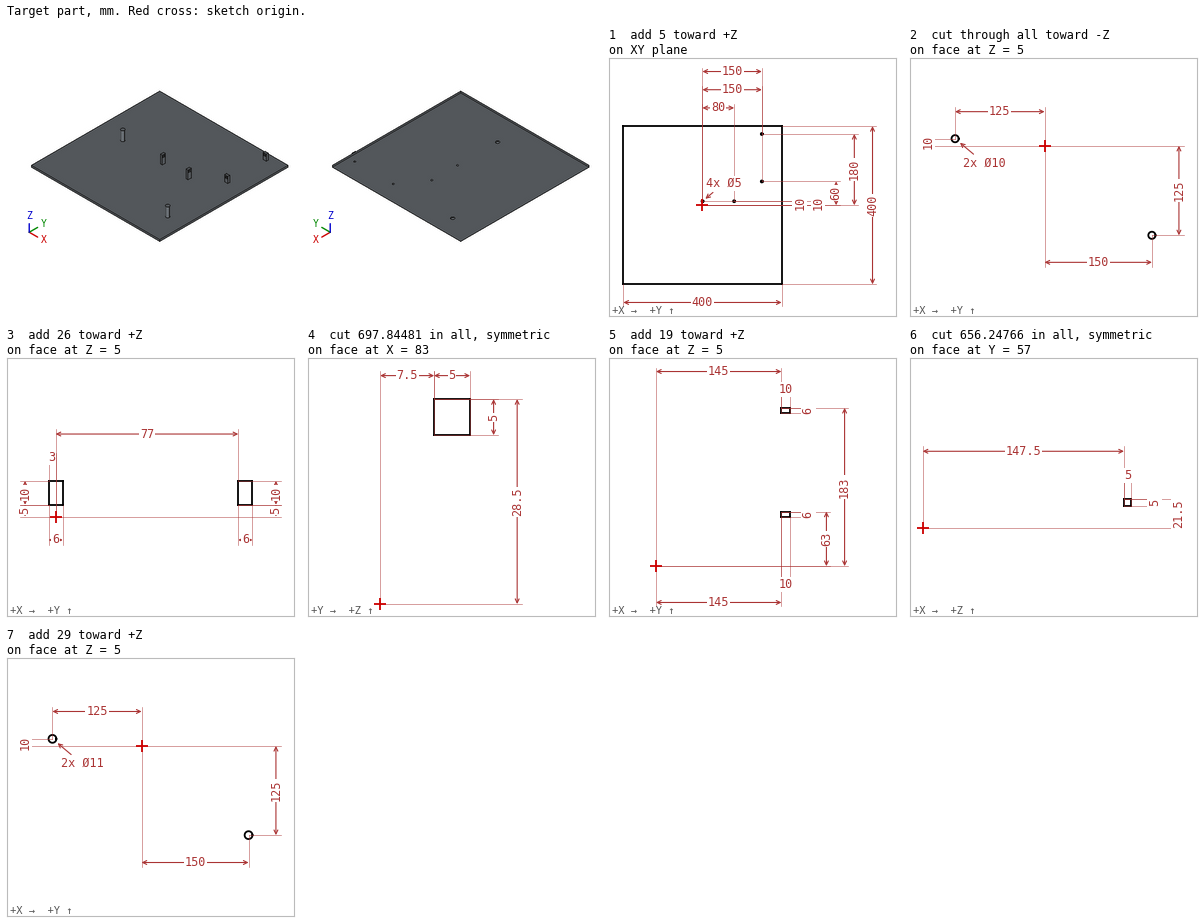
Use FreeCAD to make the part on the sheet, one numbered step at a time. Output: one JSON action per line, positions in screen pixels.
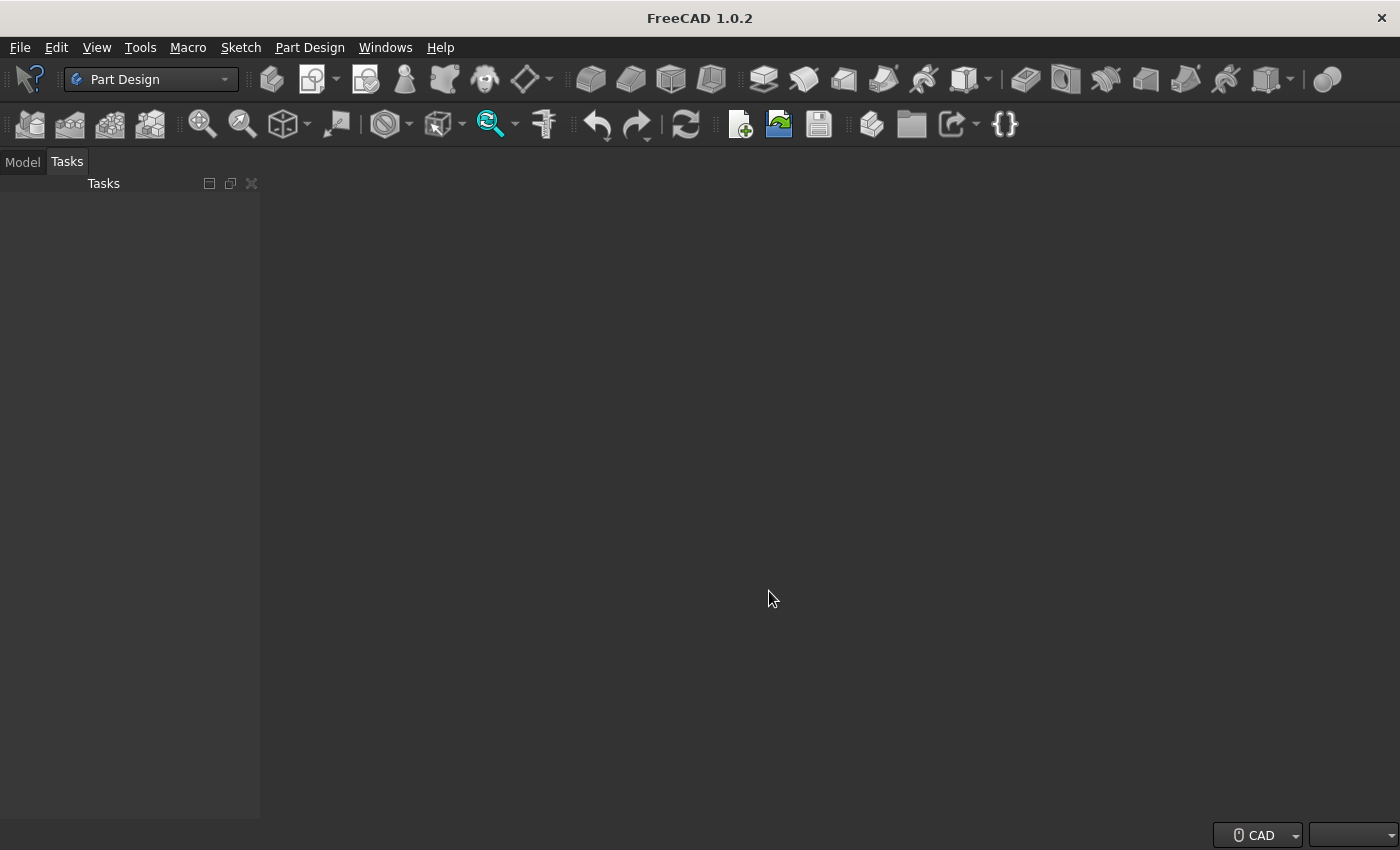
{"action": "left_click", "coordinate": [740, 124]}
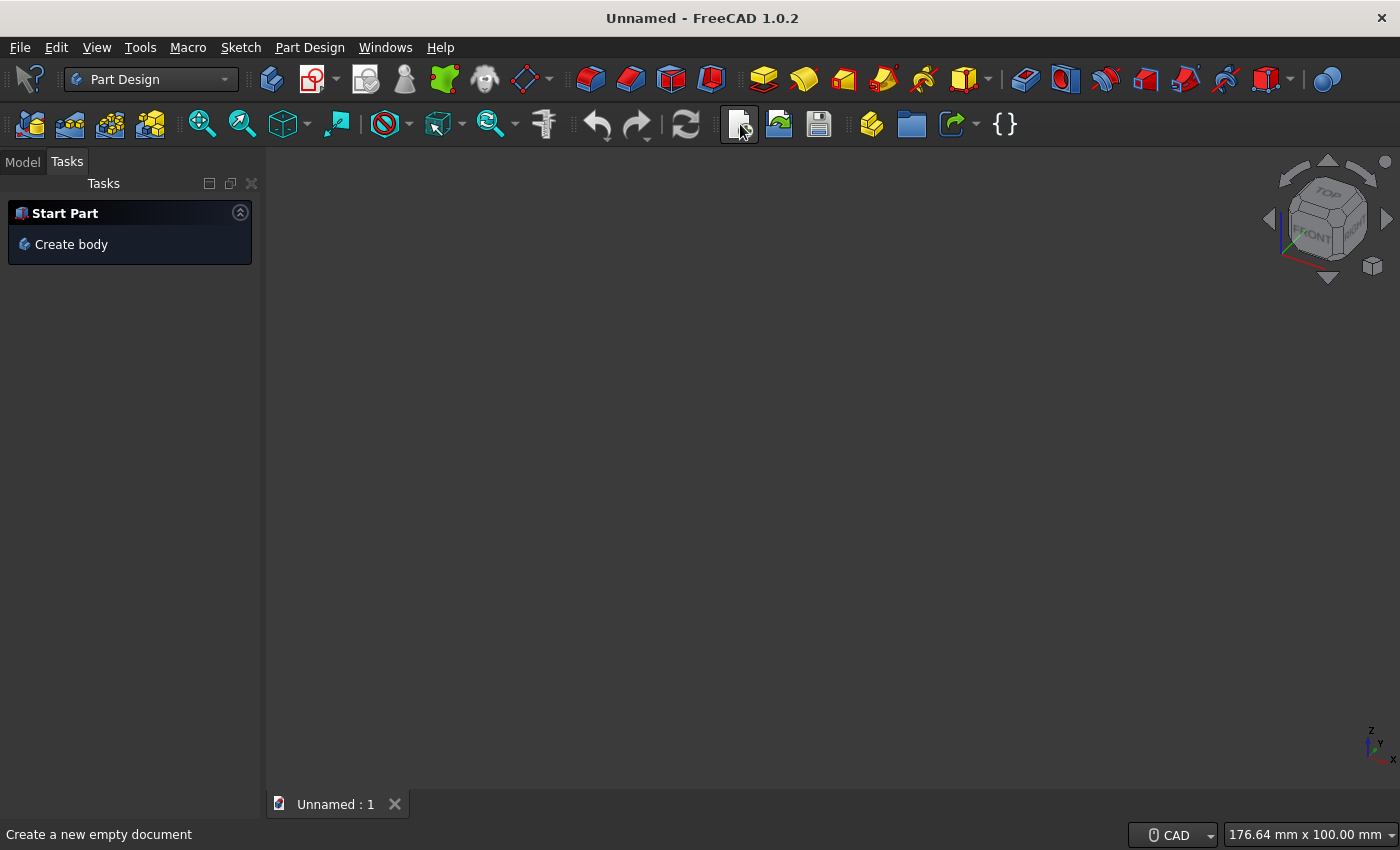
{"action": "left_click", "coordinate": [312, 80]}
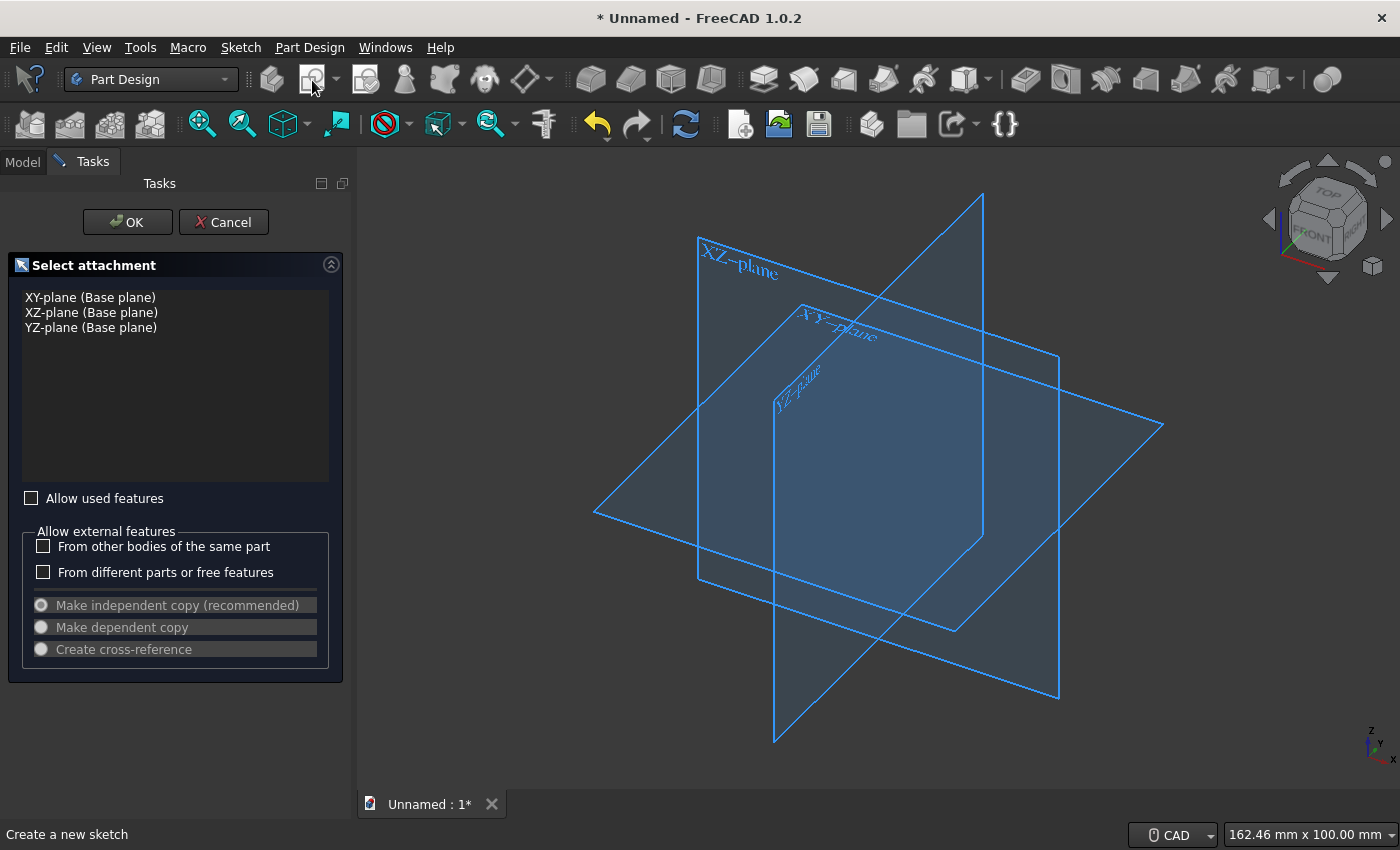
{"action": "left_click", "coordinate": [82, 298]}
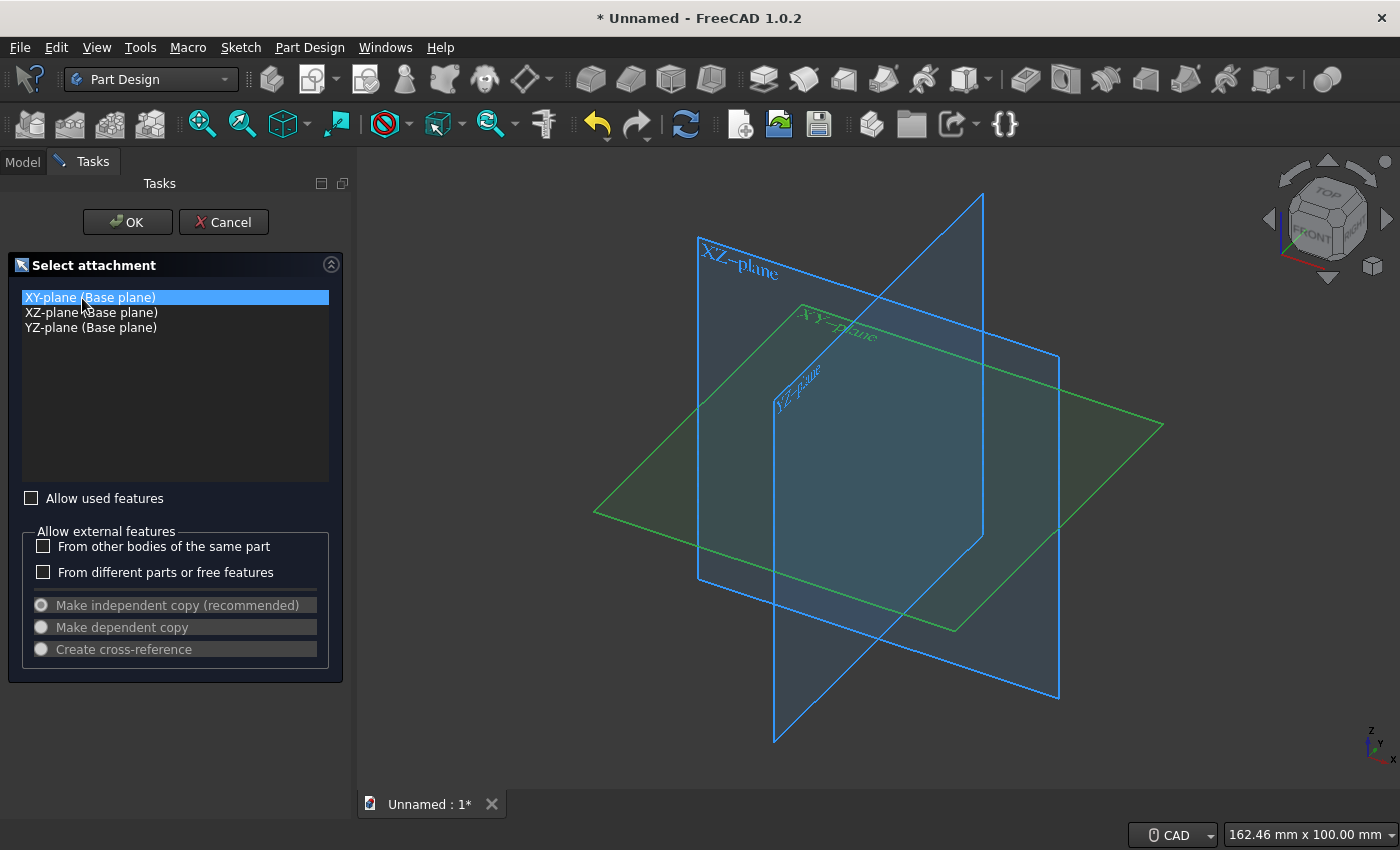
{"action": "left_click", "coordinate": [128, 222]}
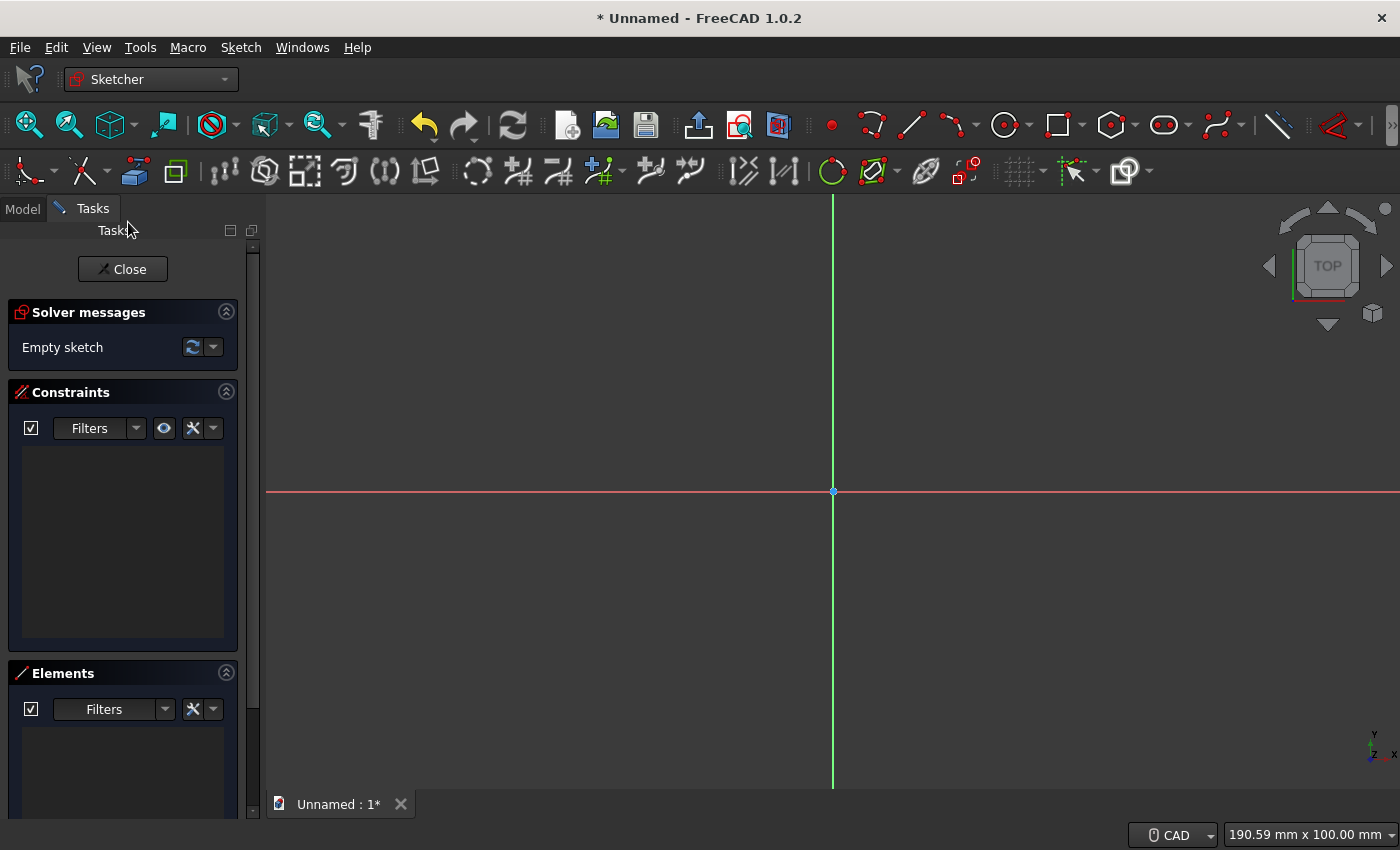
{"action": "scroll", "coordinate": [751, 492], "scroll_direction": "down", "scroll_amount": 9}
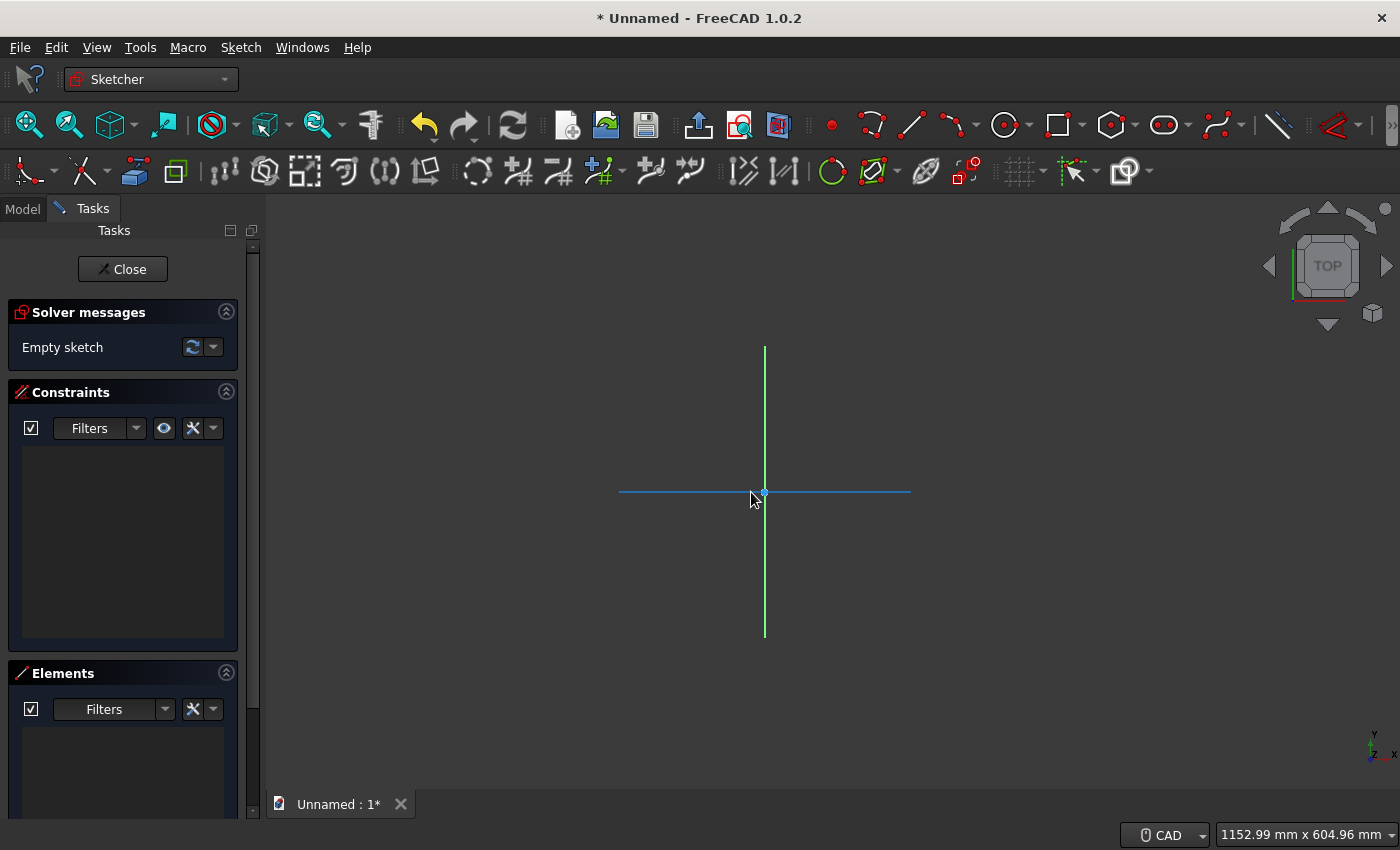
{"action": "key", "text": "g v"}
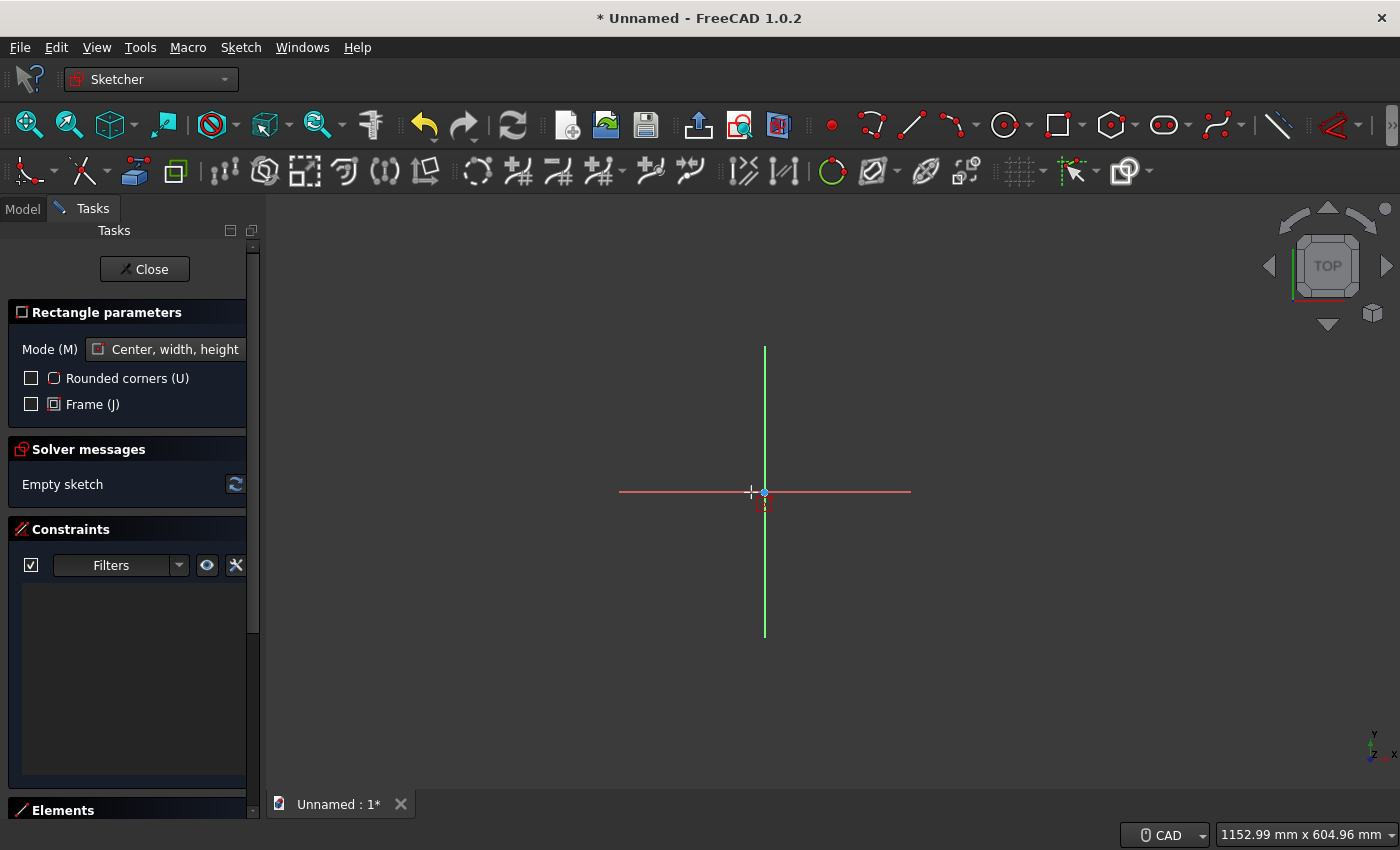
{"action": "left_click", "coordinate": [765, 492]}
{"action": "left_click", "coordinate": [962, 296]}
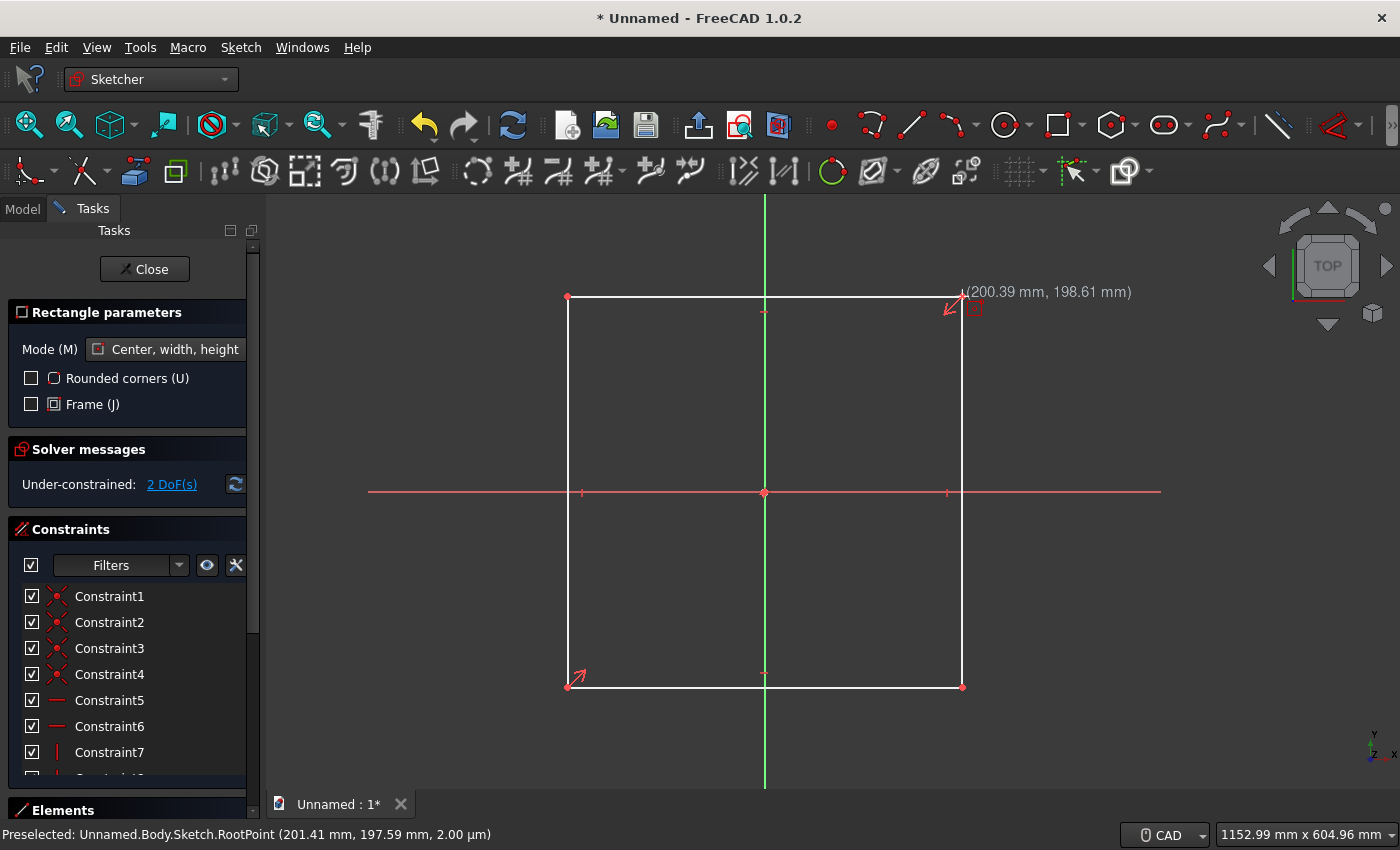
{"action": "key", "text": "g c"}